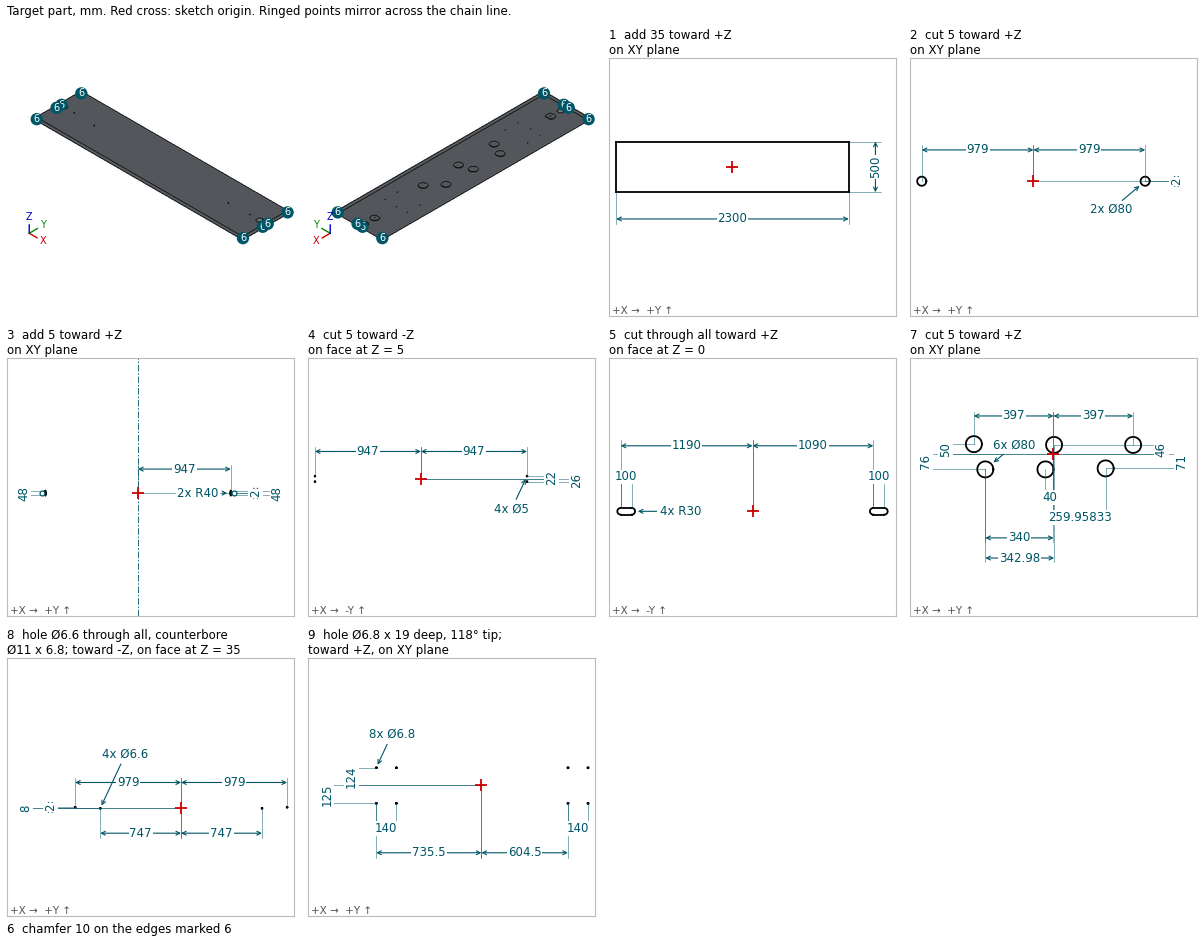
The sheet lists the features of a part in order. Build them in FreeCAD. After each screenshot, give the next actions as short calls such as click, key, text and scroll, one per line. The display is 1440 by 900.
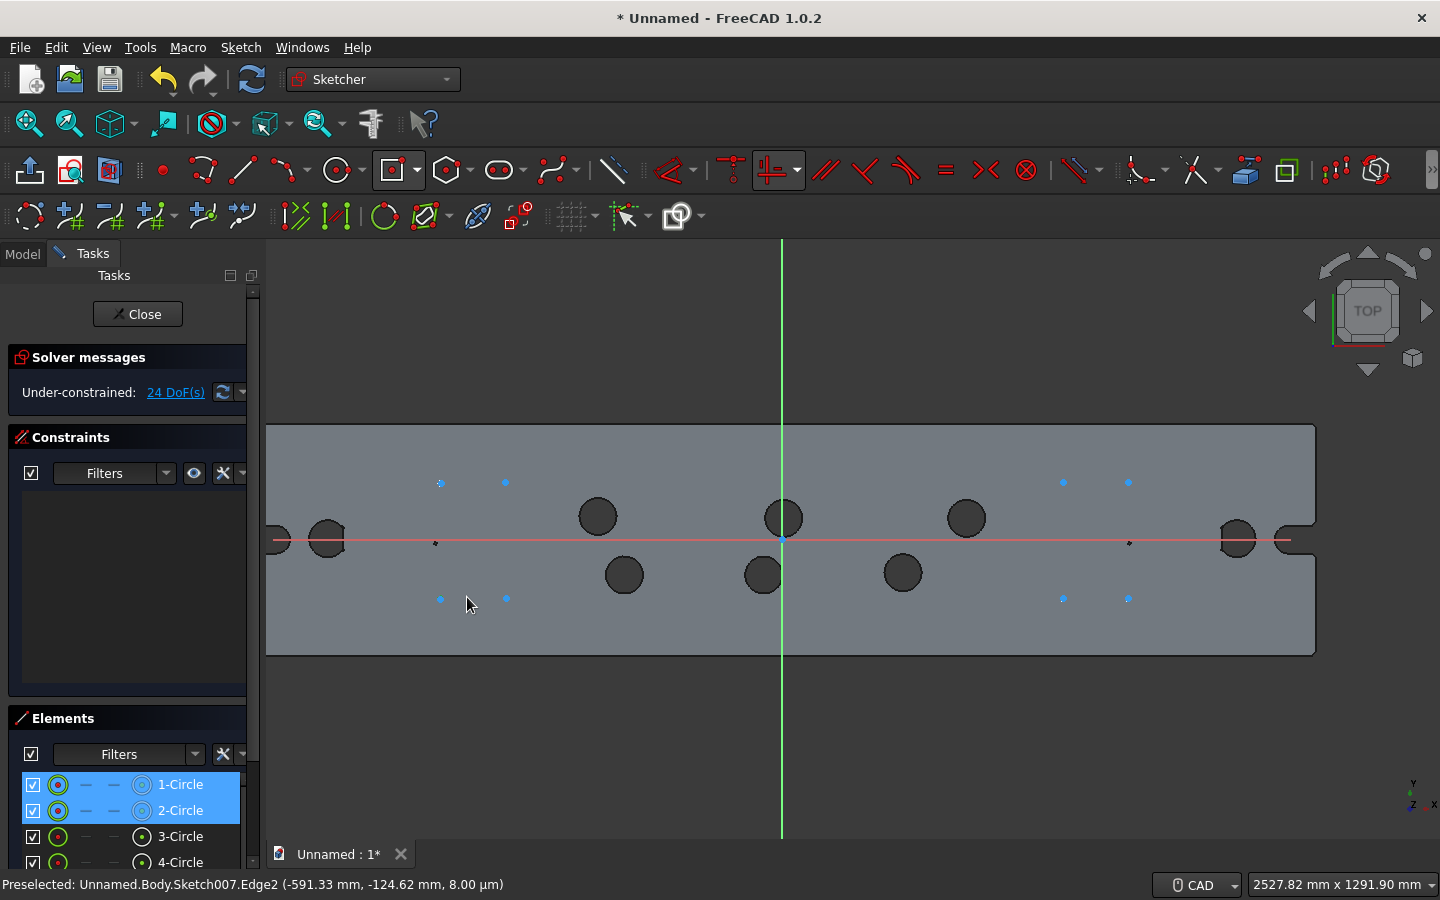
scroll(443, 482, up, 9)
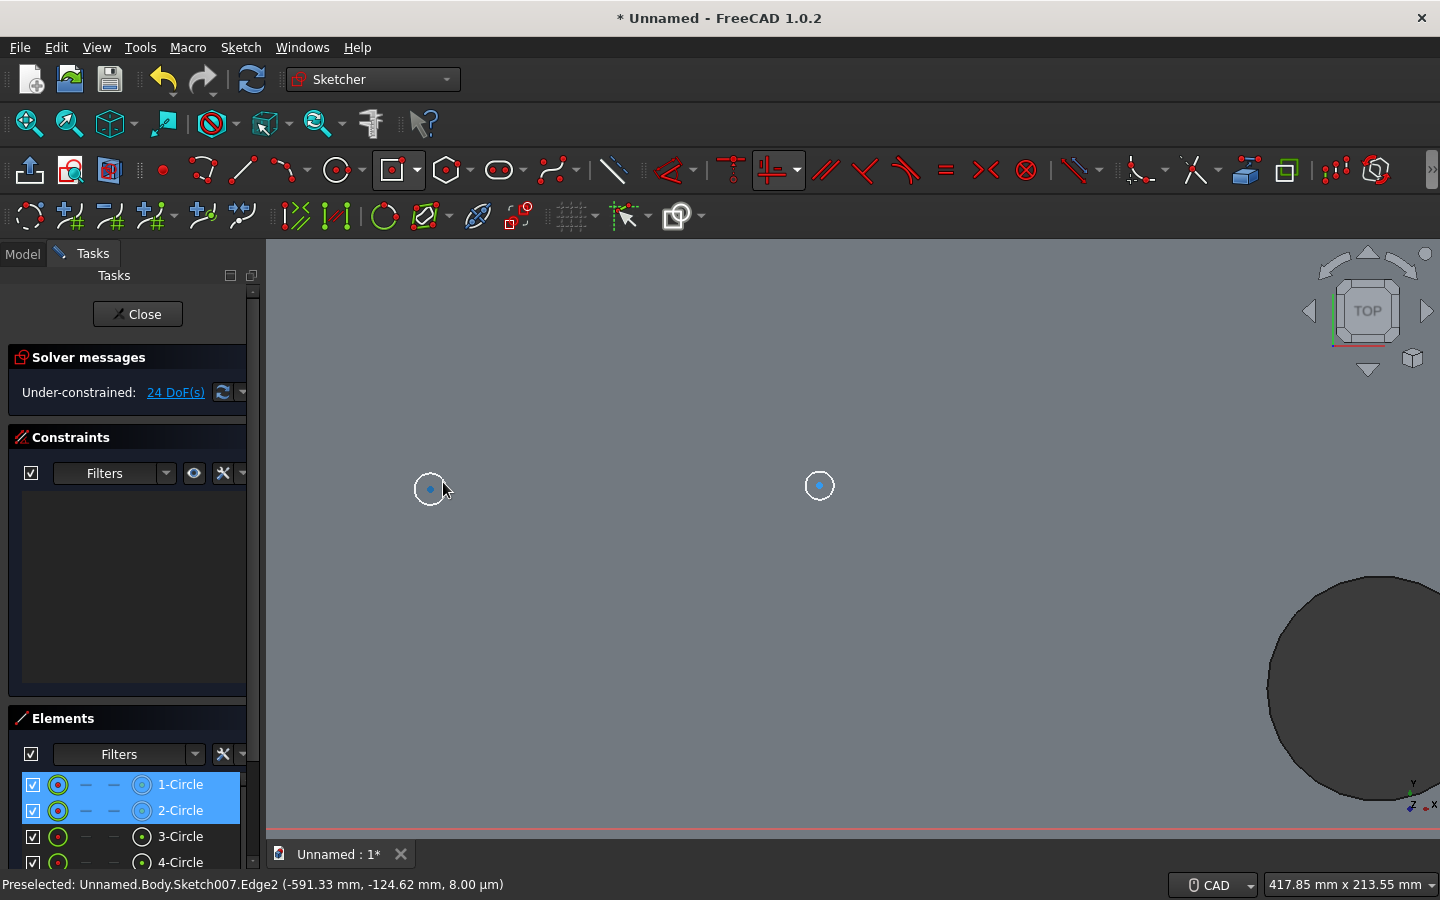
click(441, 478)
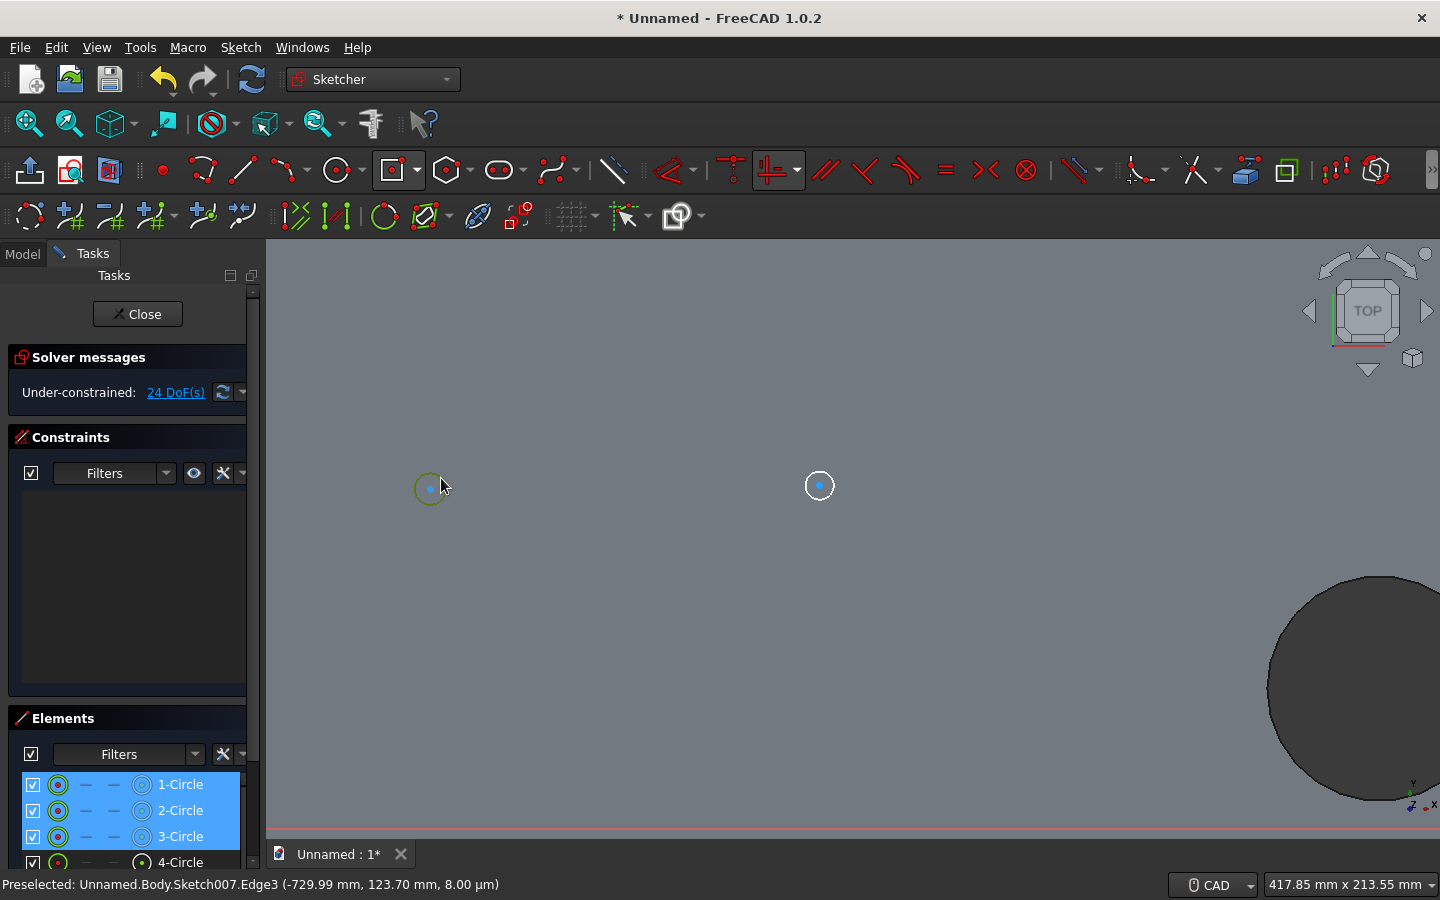
click(830, 476)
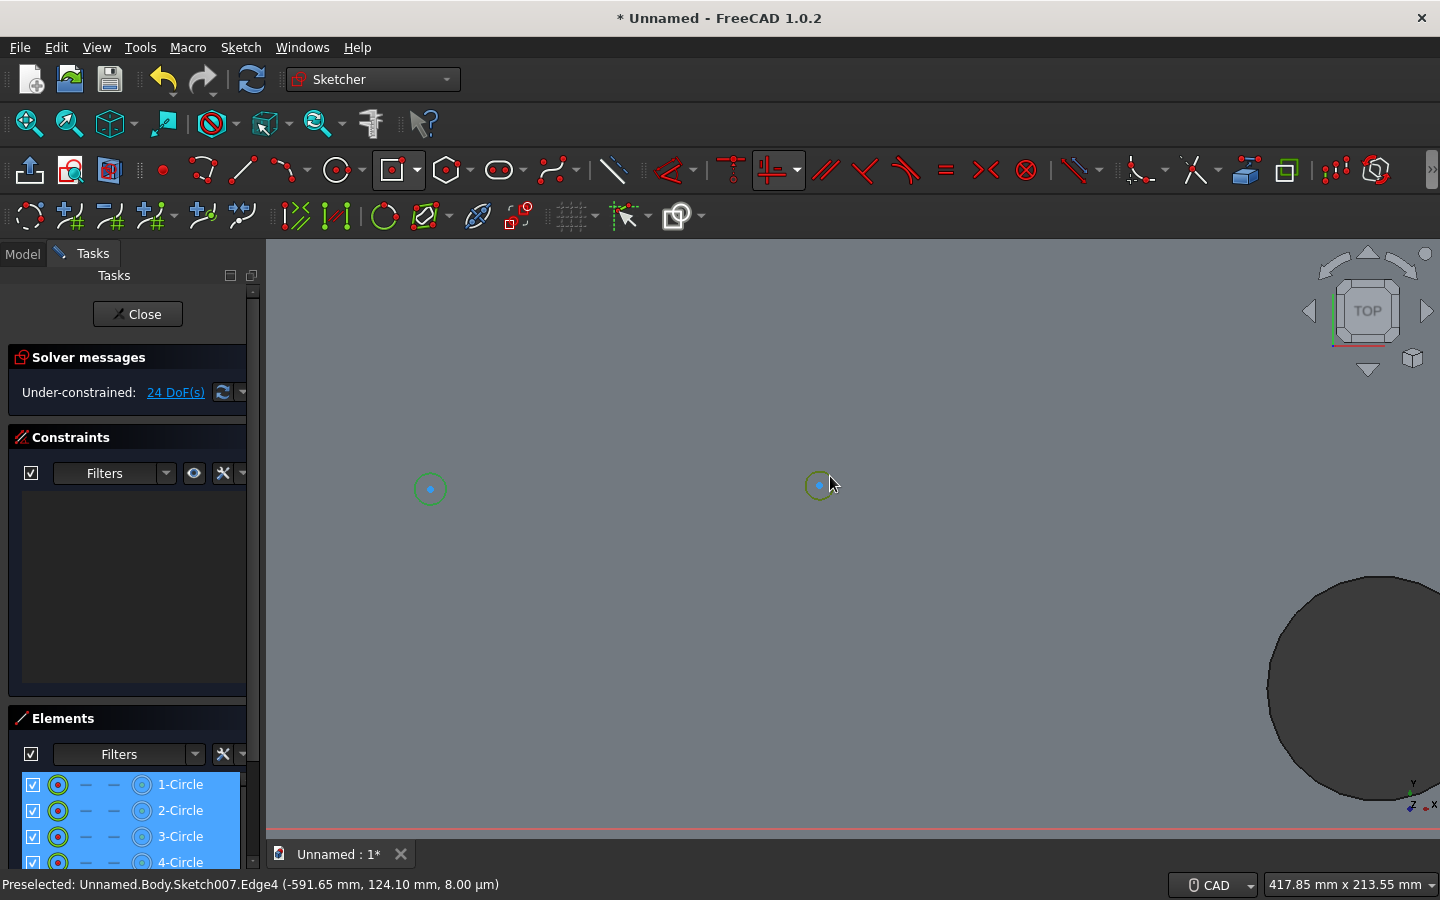
scroll(443, 481, down, 9)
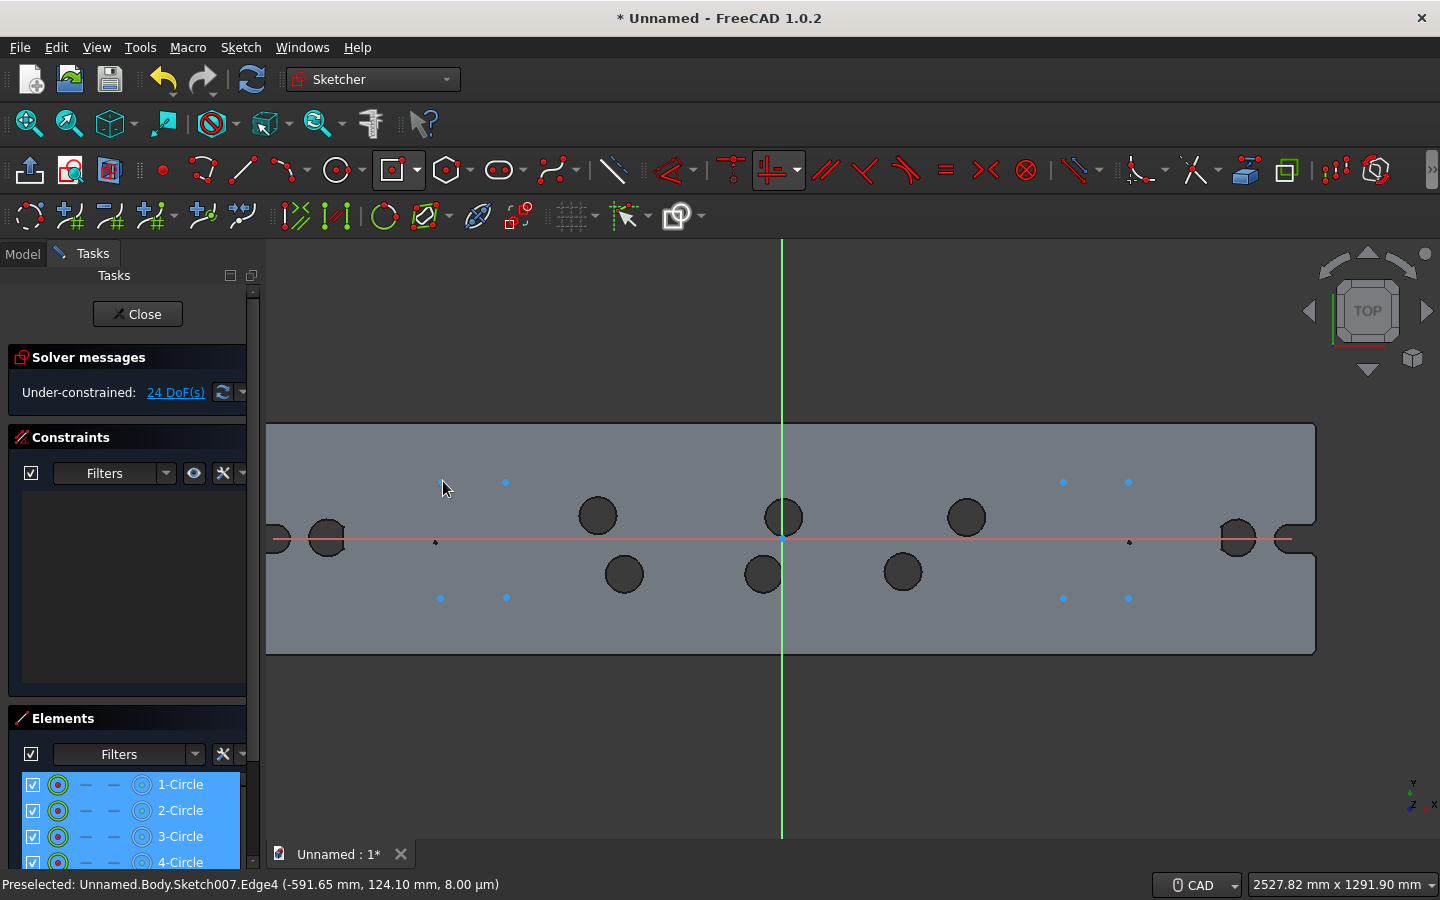
scroll(1065, 596, up, 9)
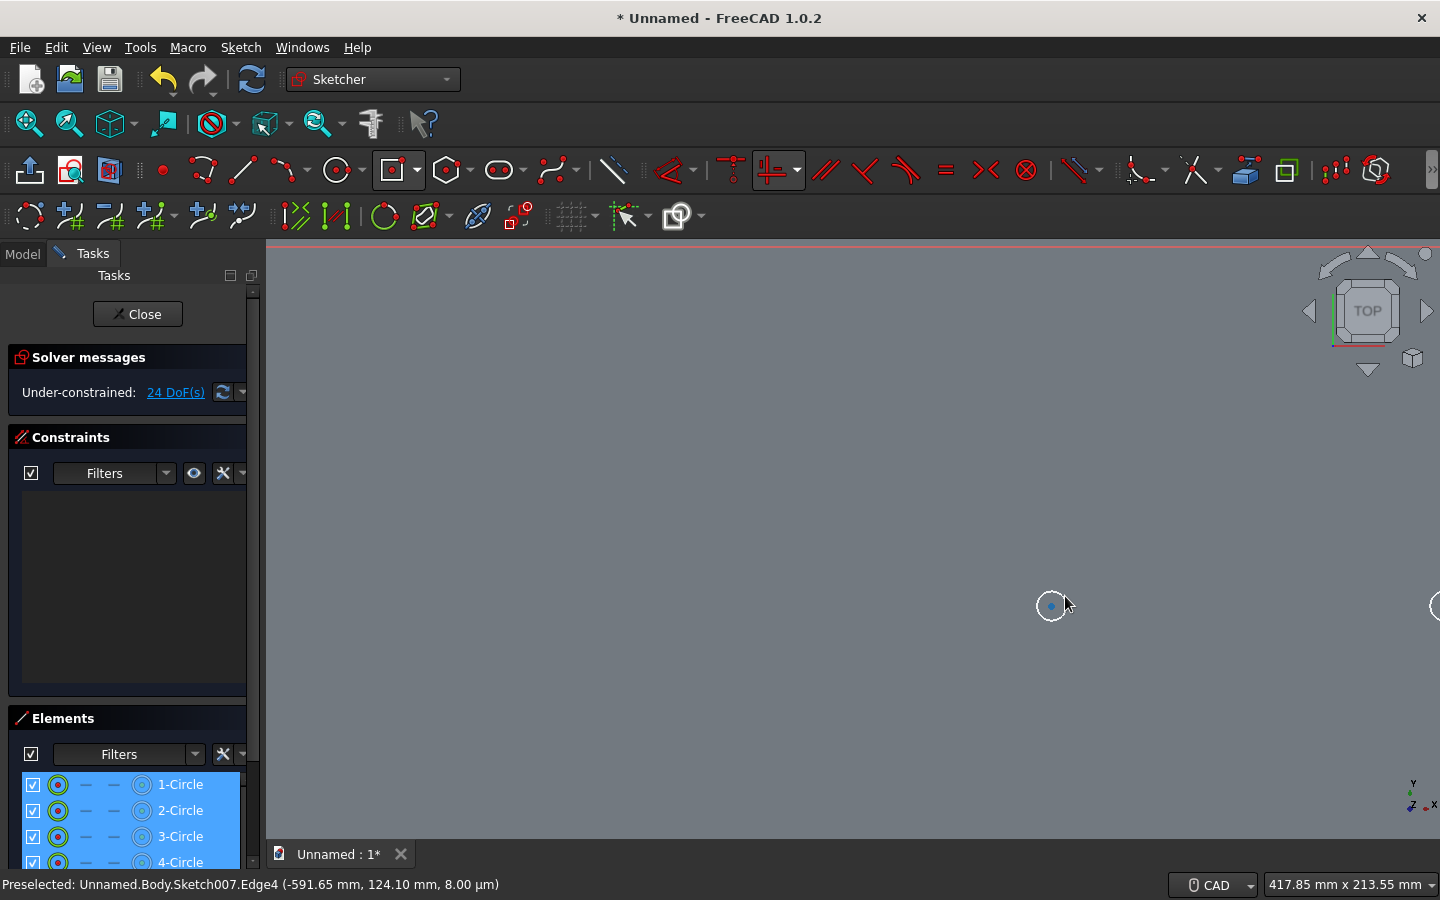
click(1062, 596)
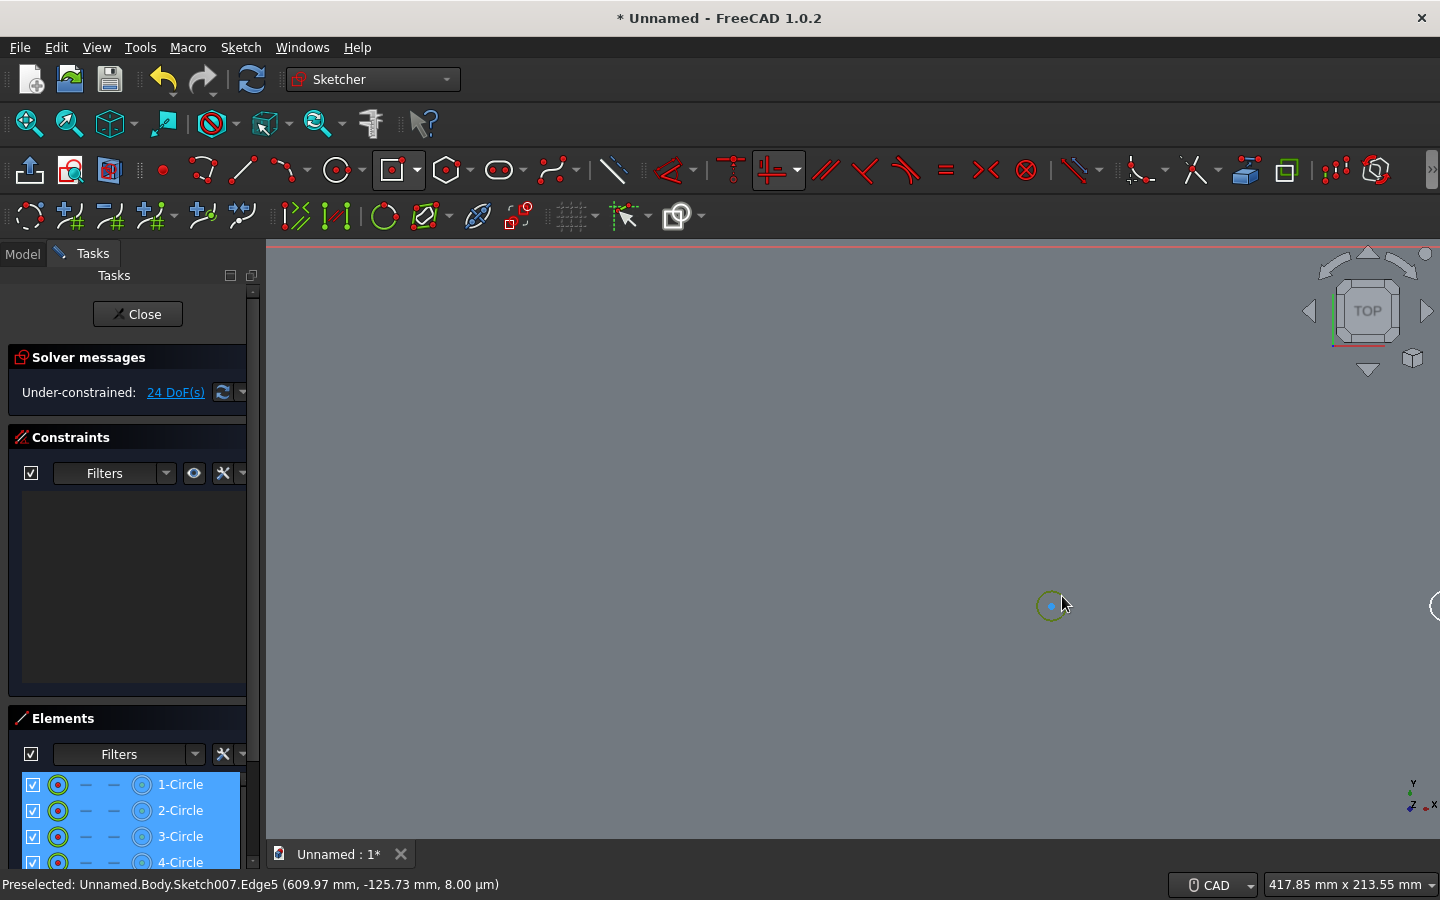
scroll(1066, 596, down, 9)